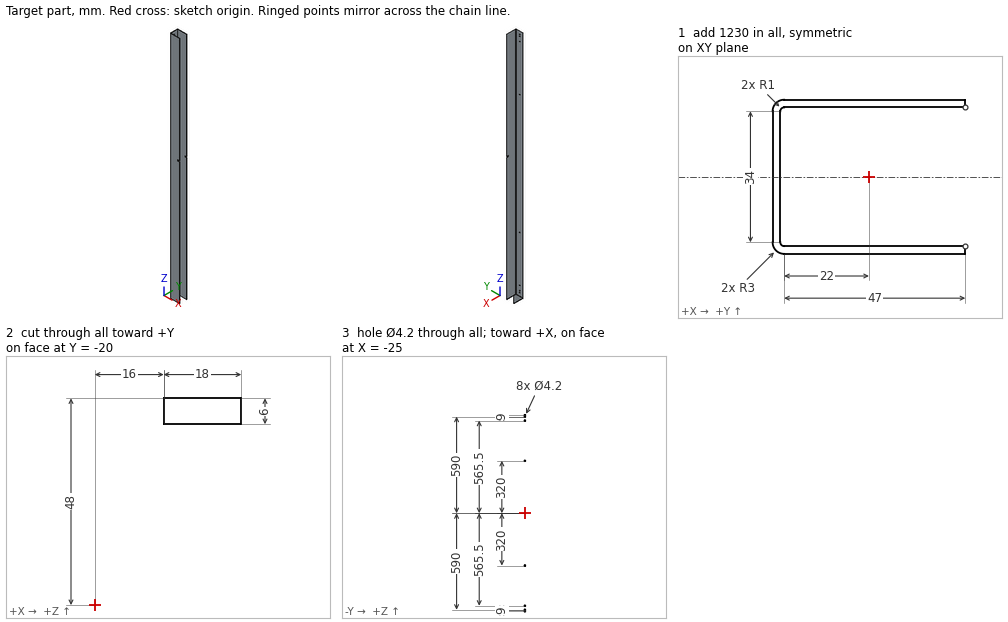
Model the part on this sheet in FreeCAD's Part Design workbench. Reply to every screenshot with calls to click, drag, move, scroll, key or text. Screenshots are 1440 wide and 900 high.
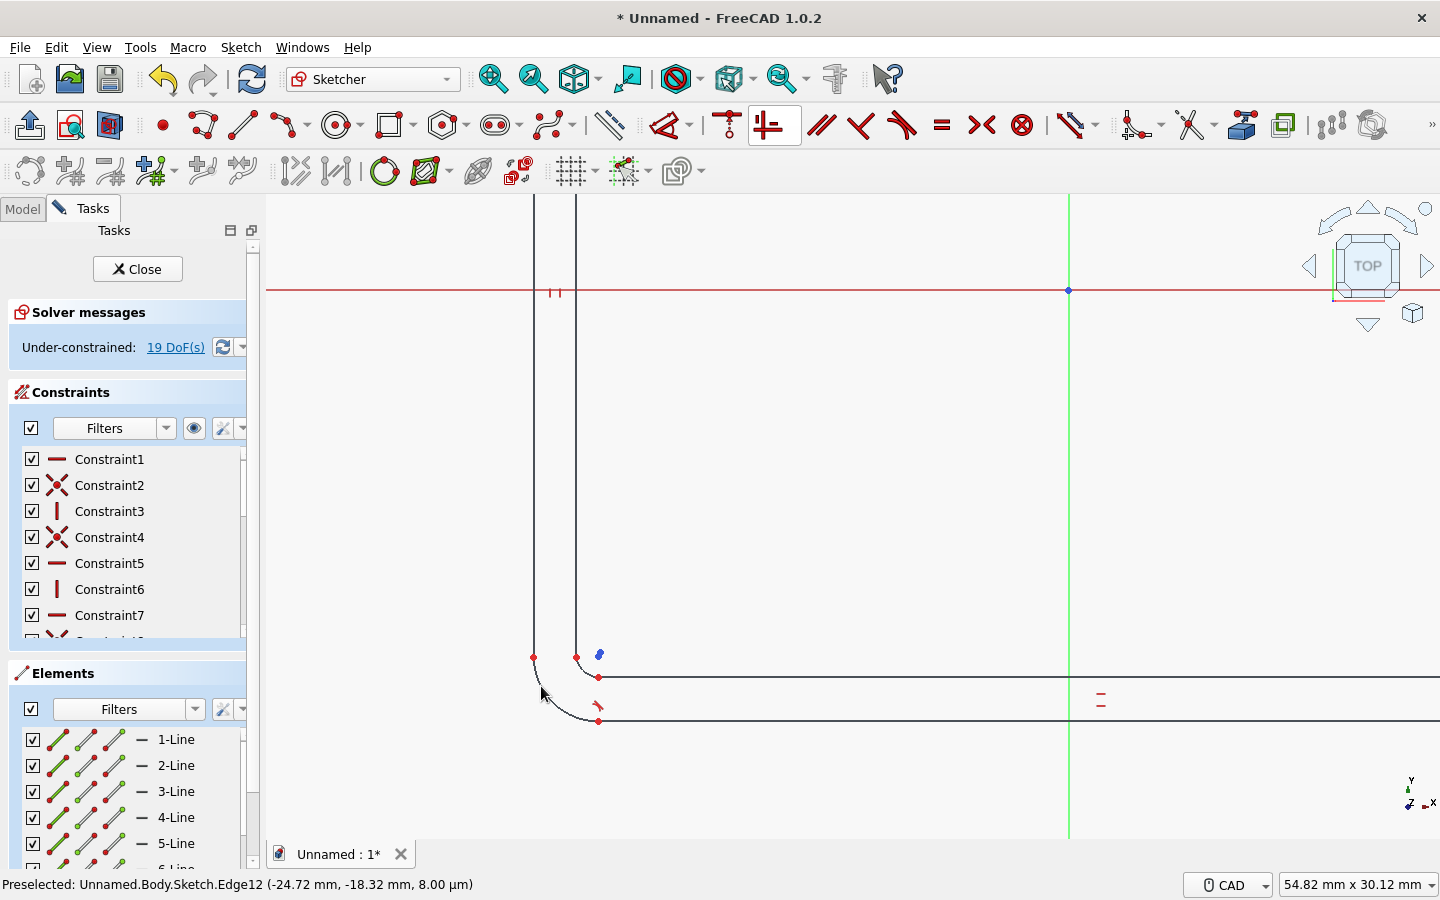
click(900, 677)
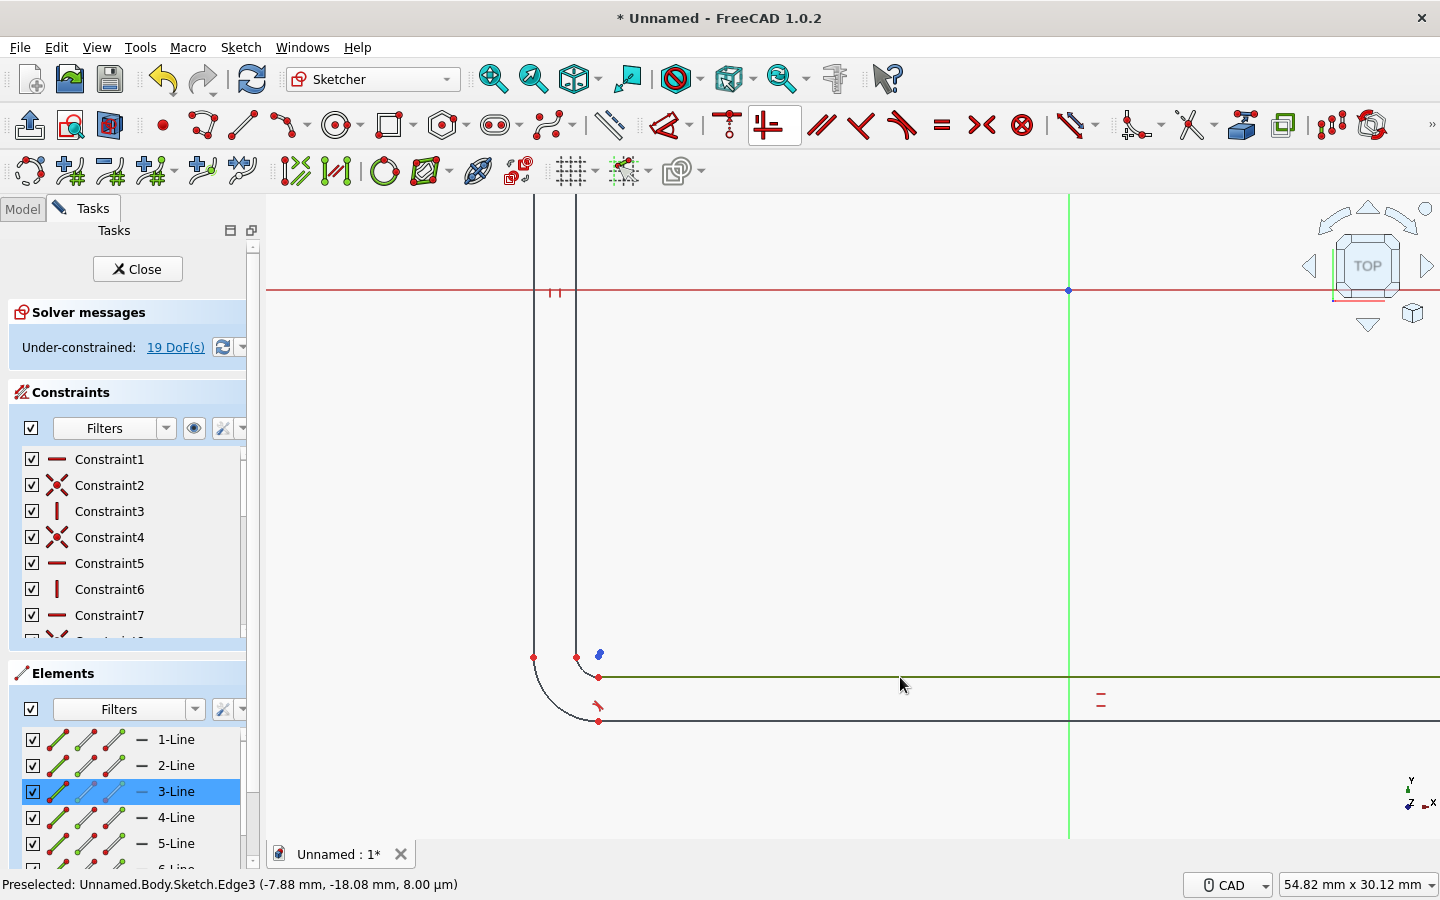
scroll(580, 666, up, 2)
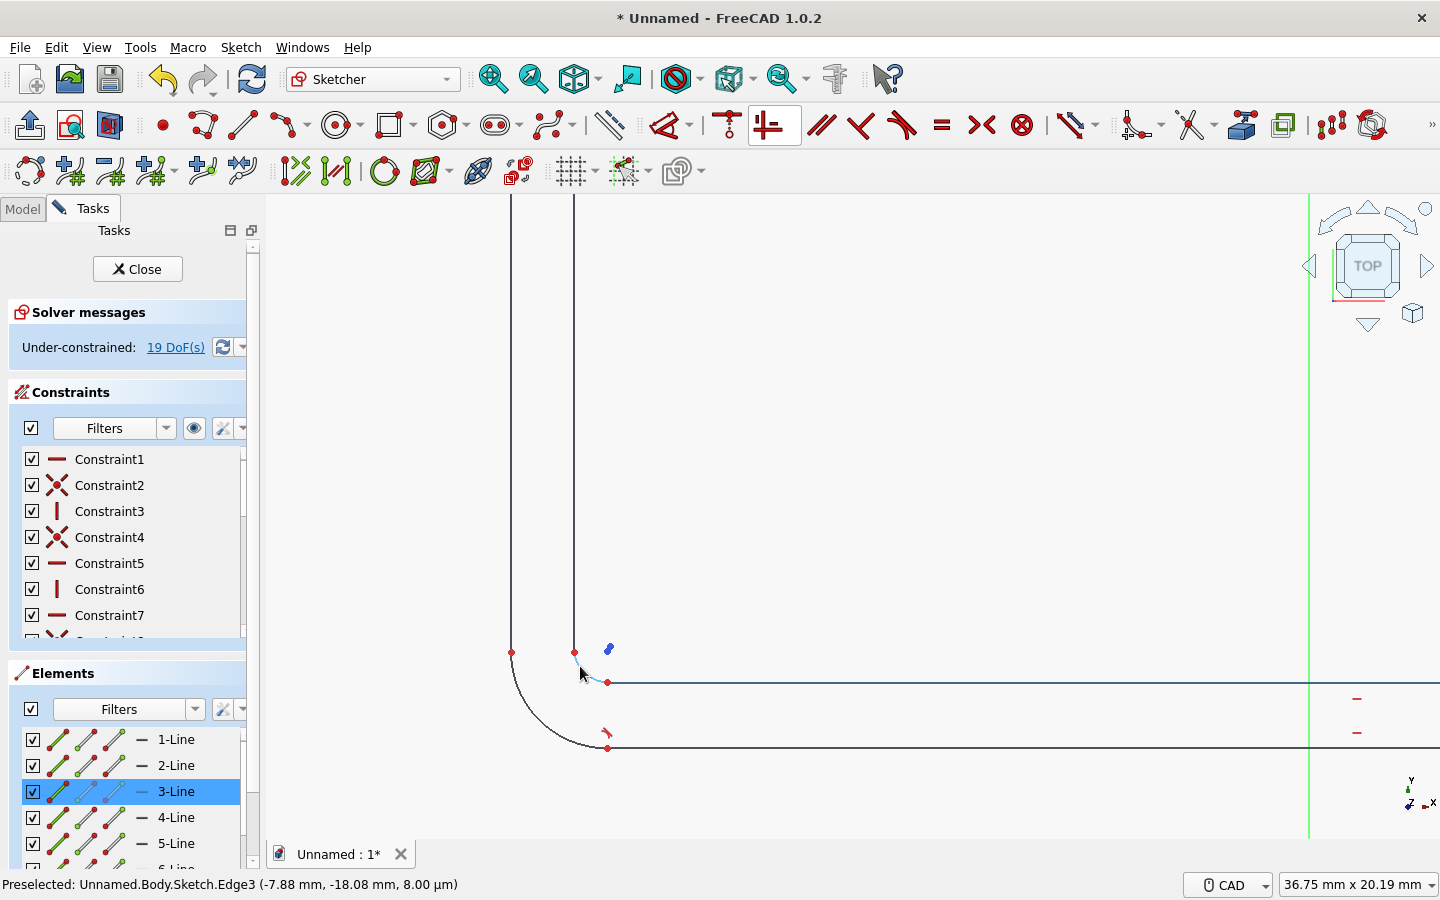
click(579, 666)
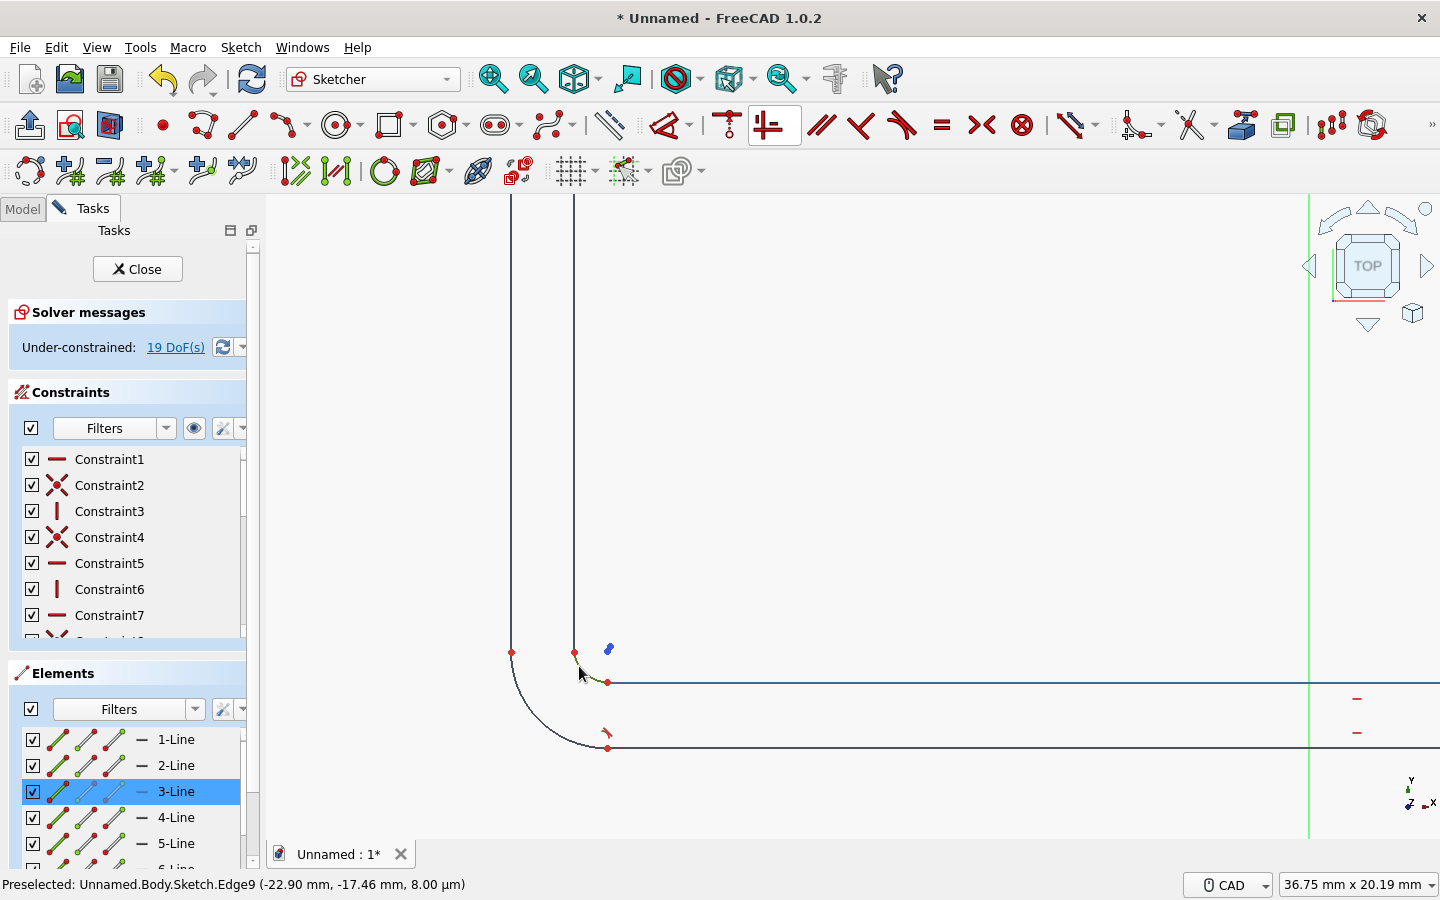
key(t)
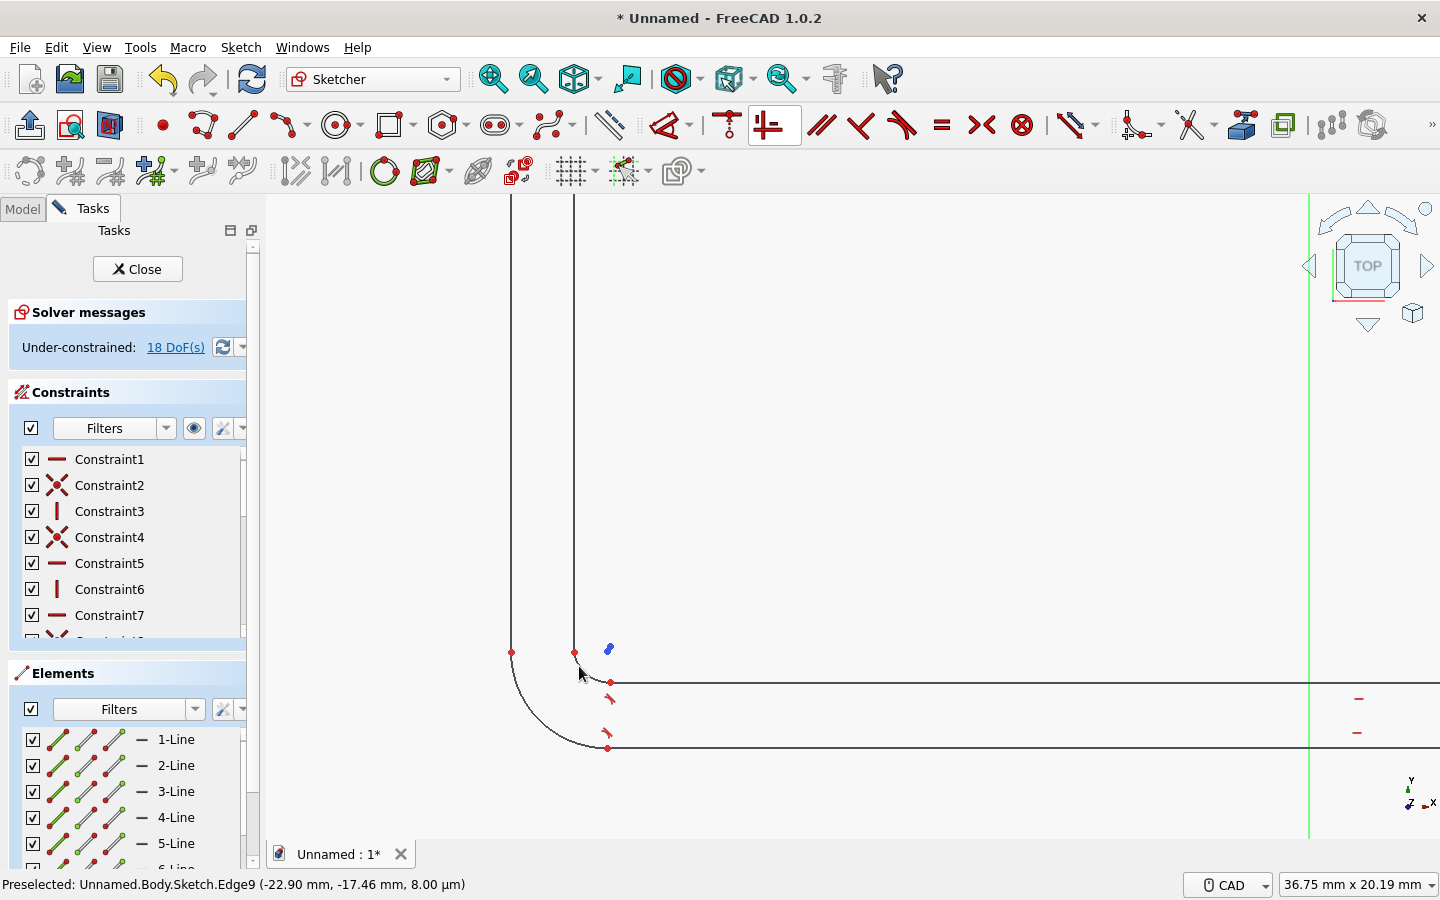
click(574, 326)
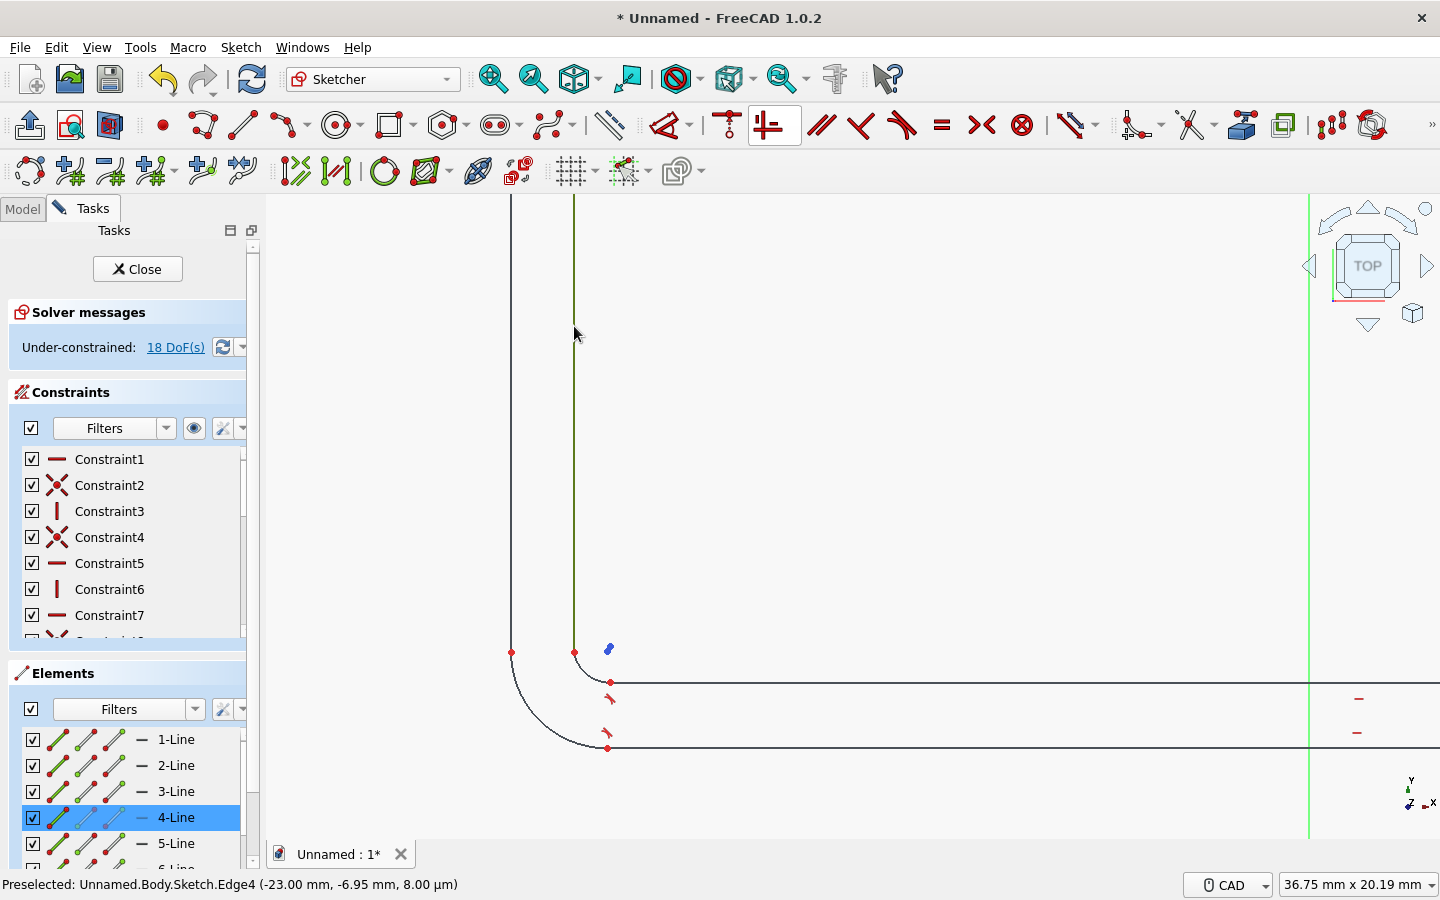
click(580, 667)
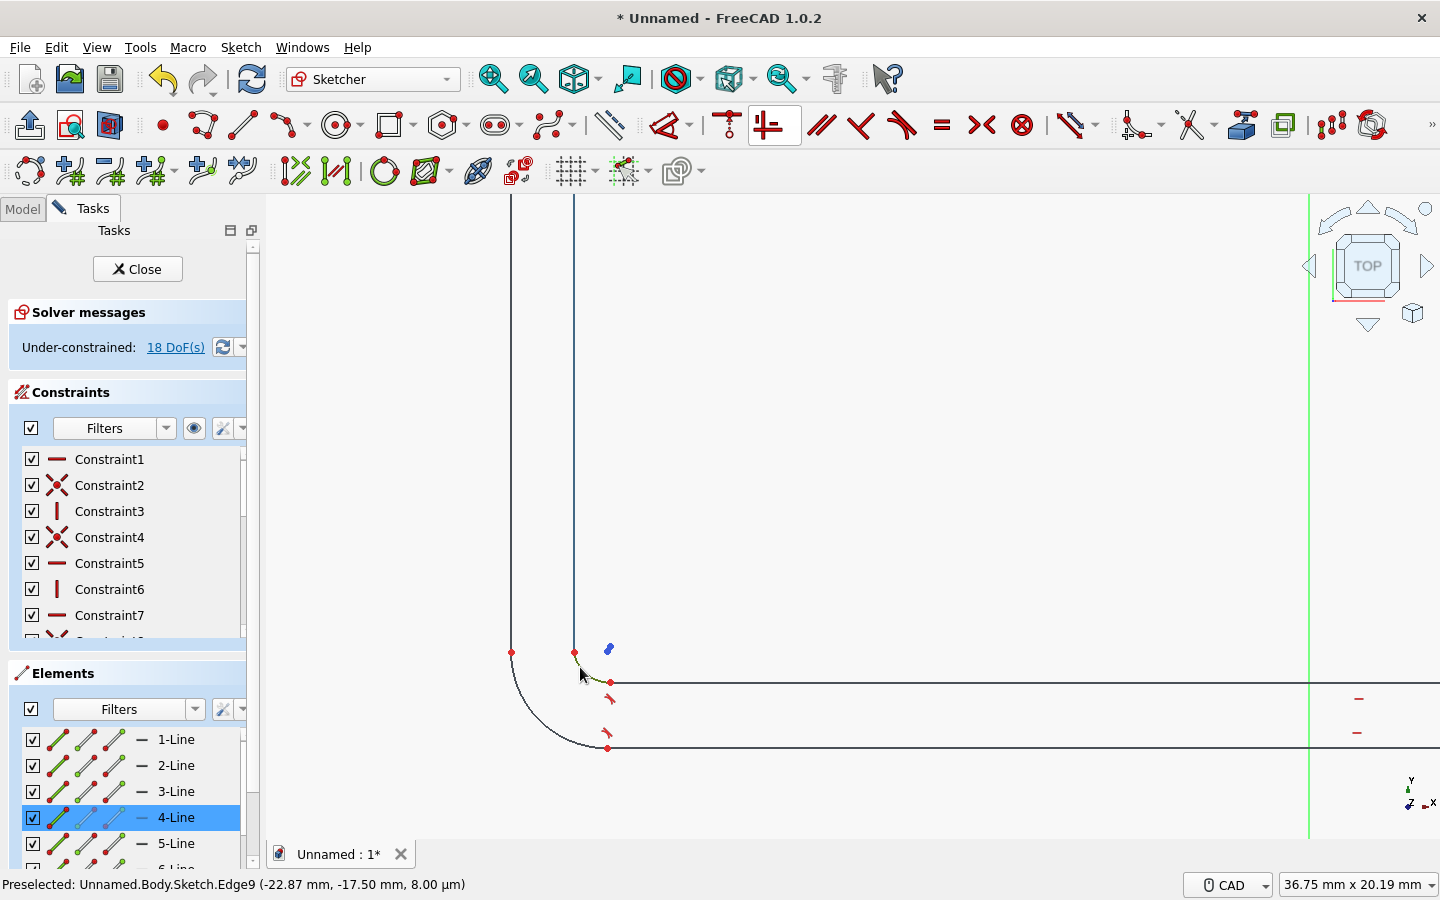
click(902, 126)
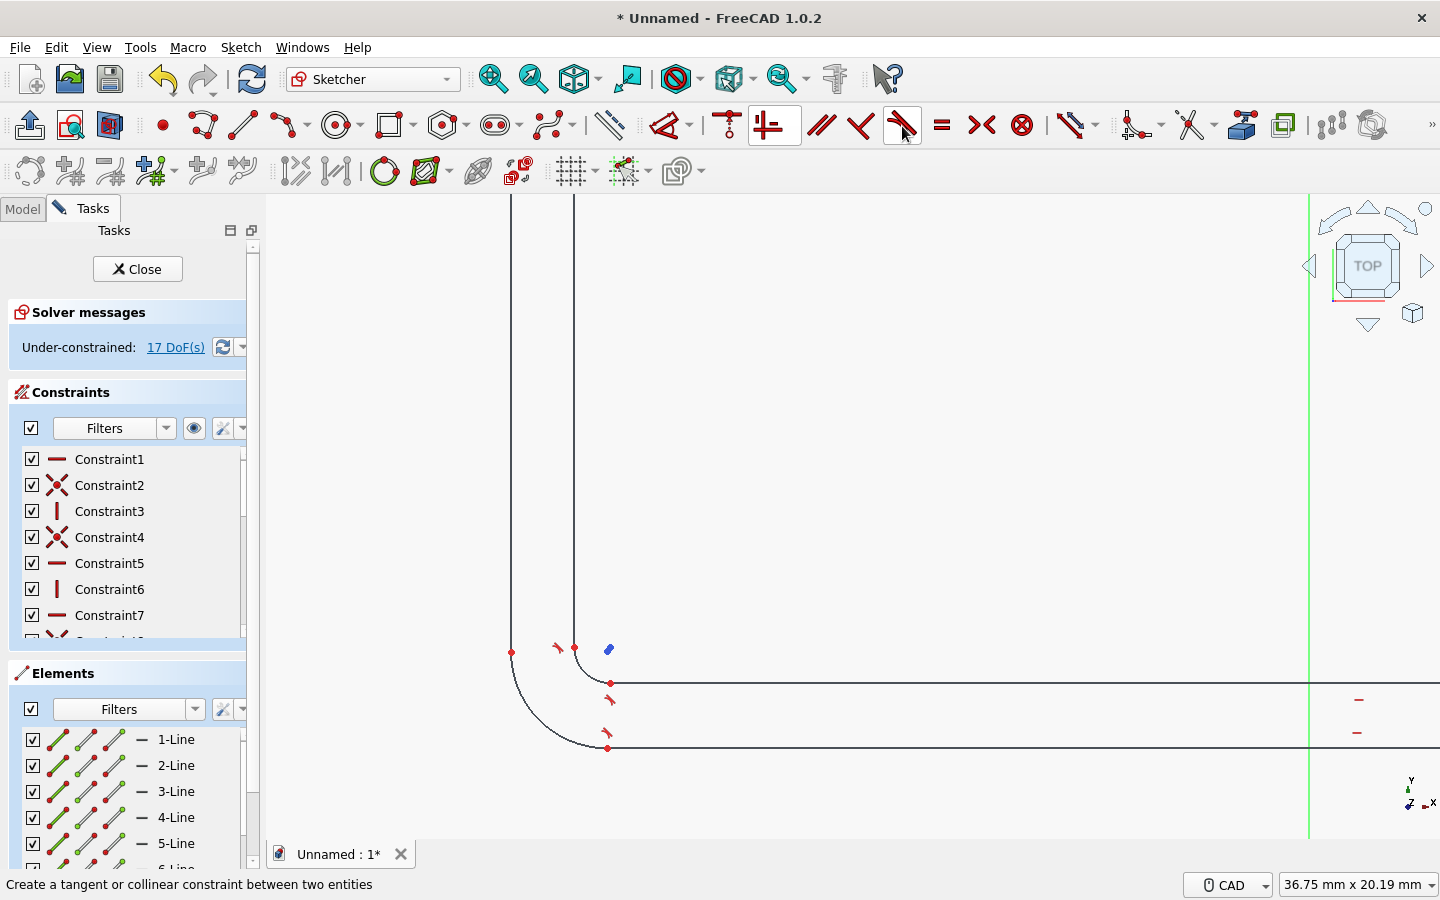
click(574, 322)